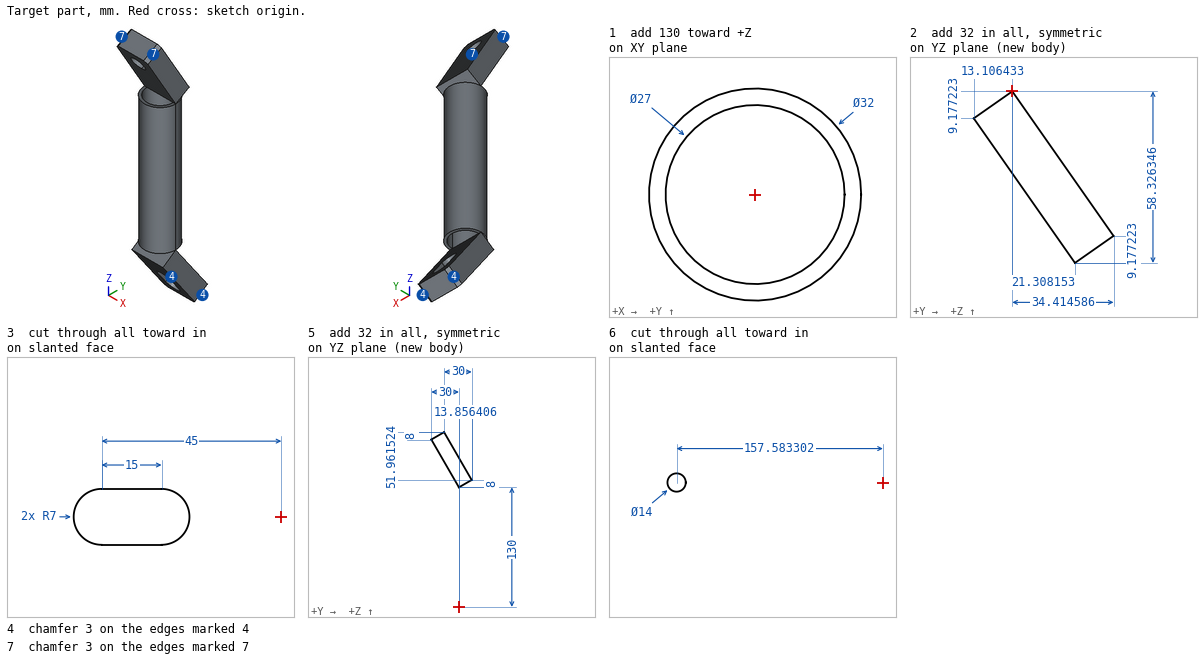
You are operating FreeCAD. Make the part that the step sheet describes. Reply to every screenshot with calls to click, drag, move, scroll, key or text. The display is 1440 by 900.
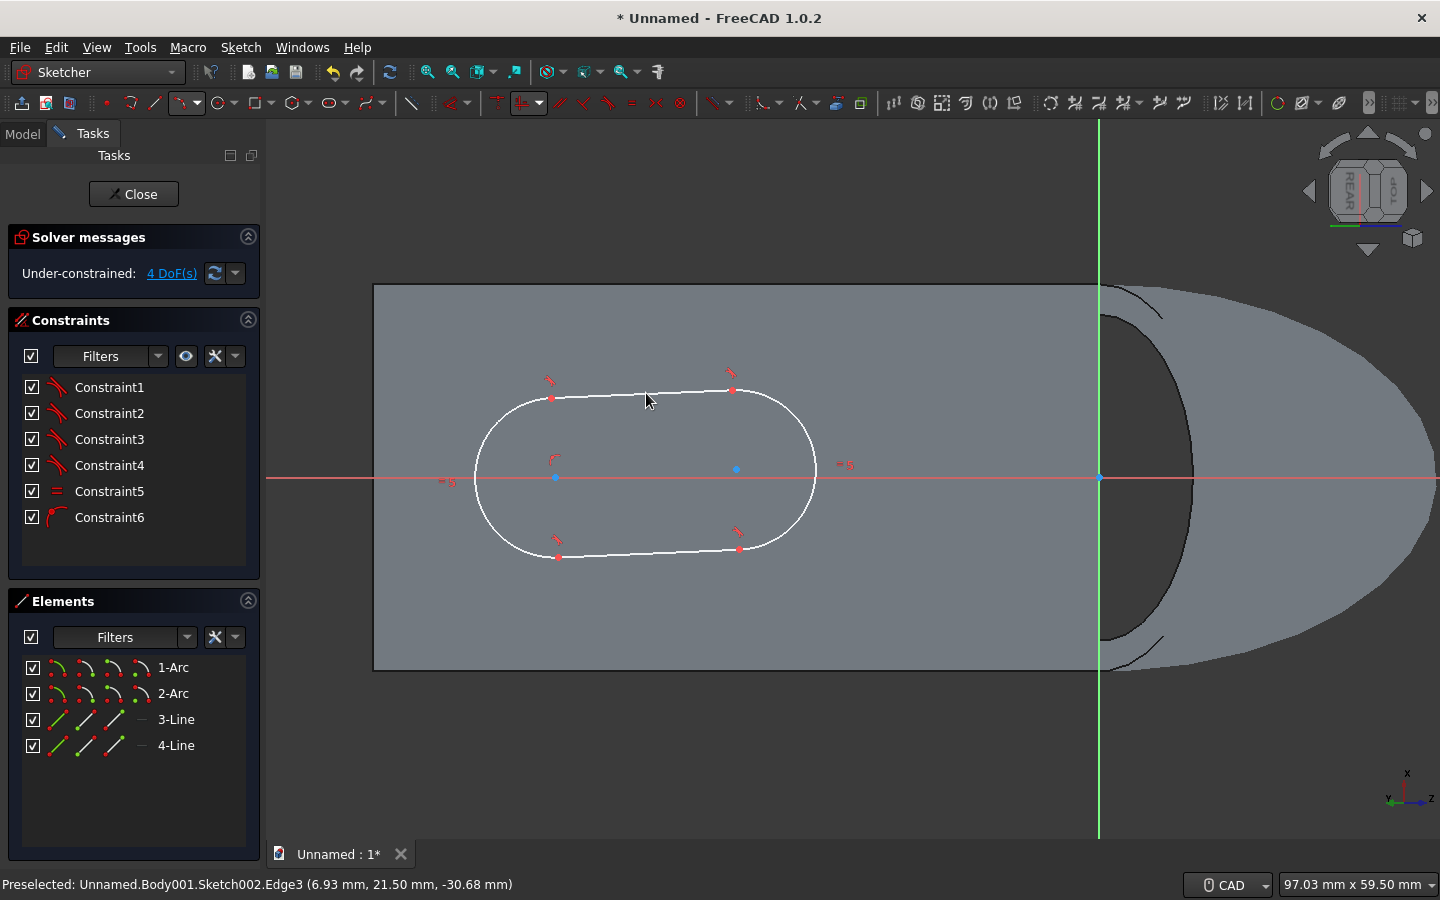
click(606, 396)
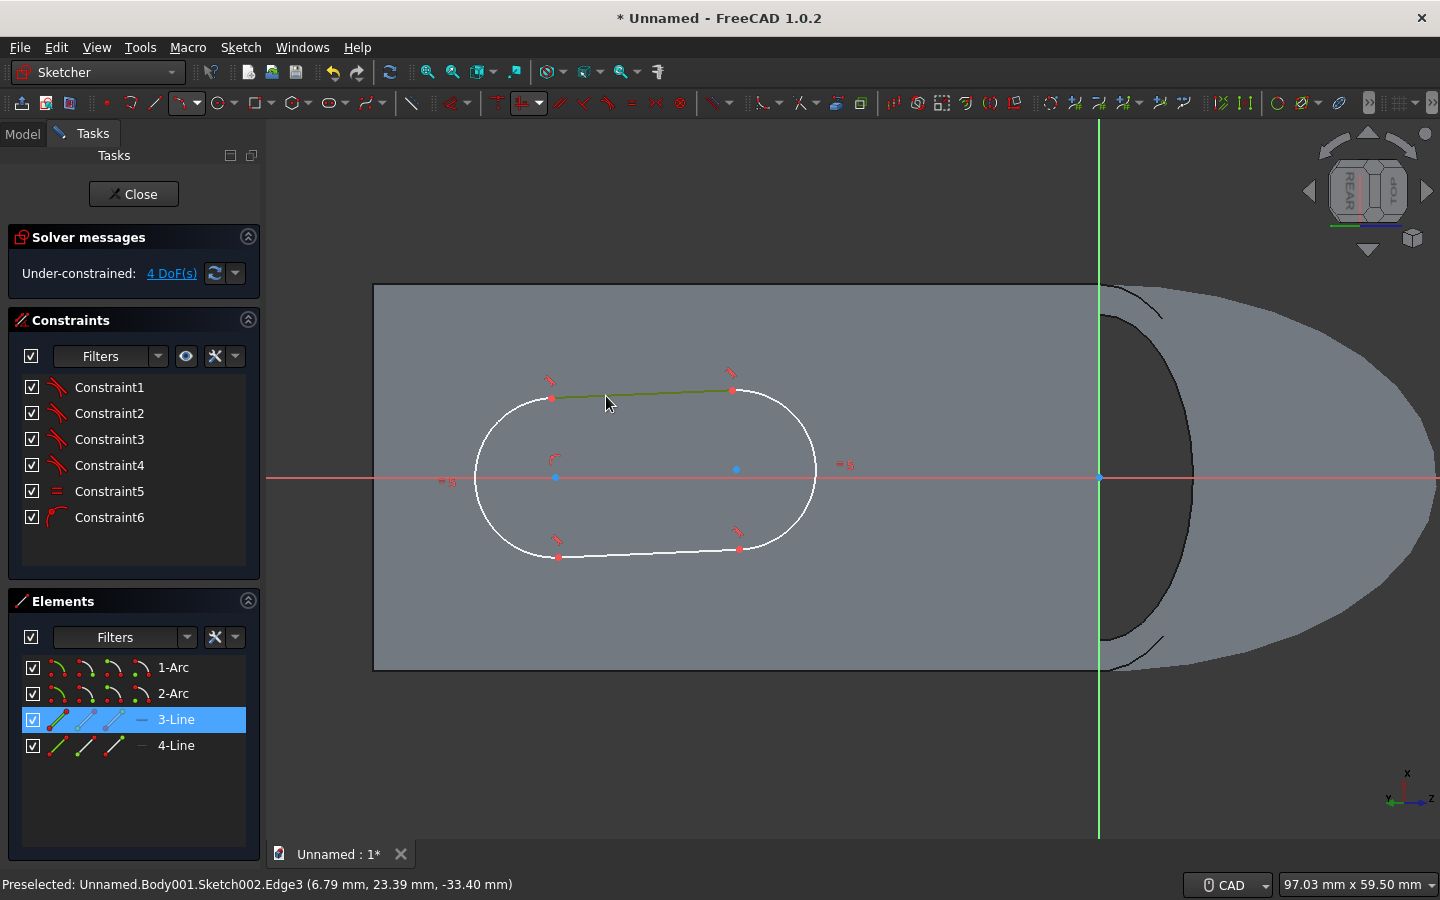
key(h)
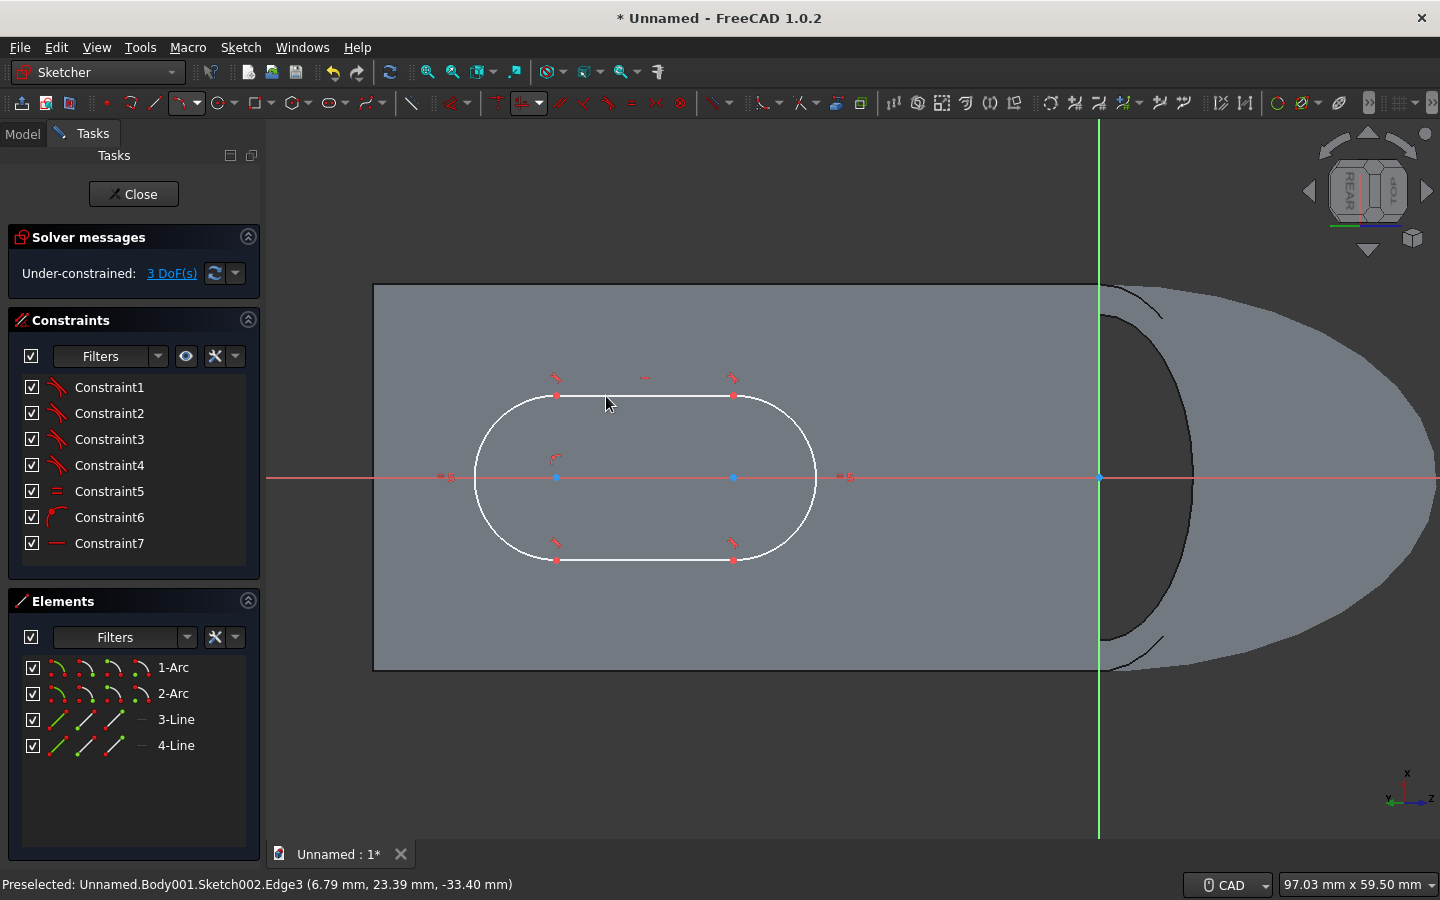
click(450, 104)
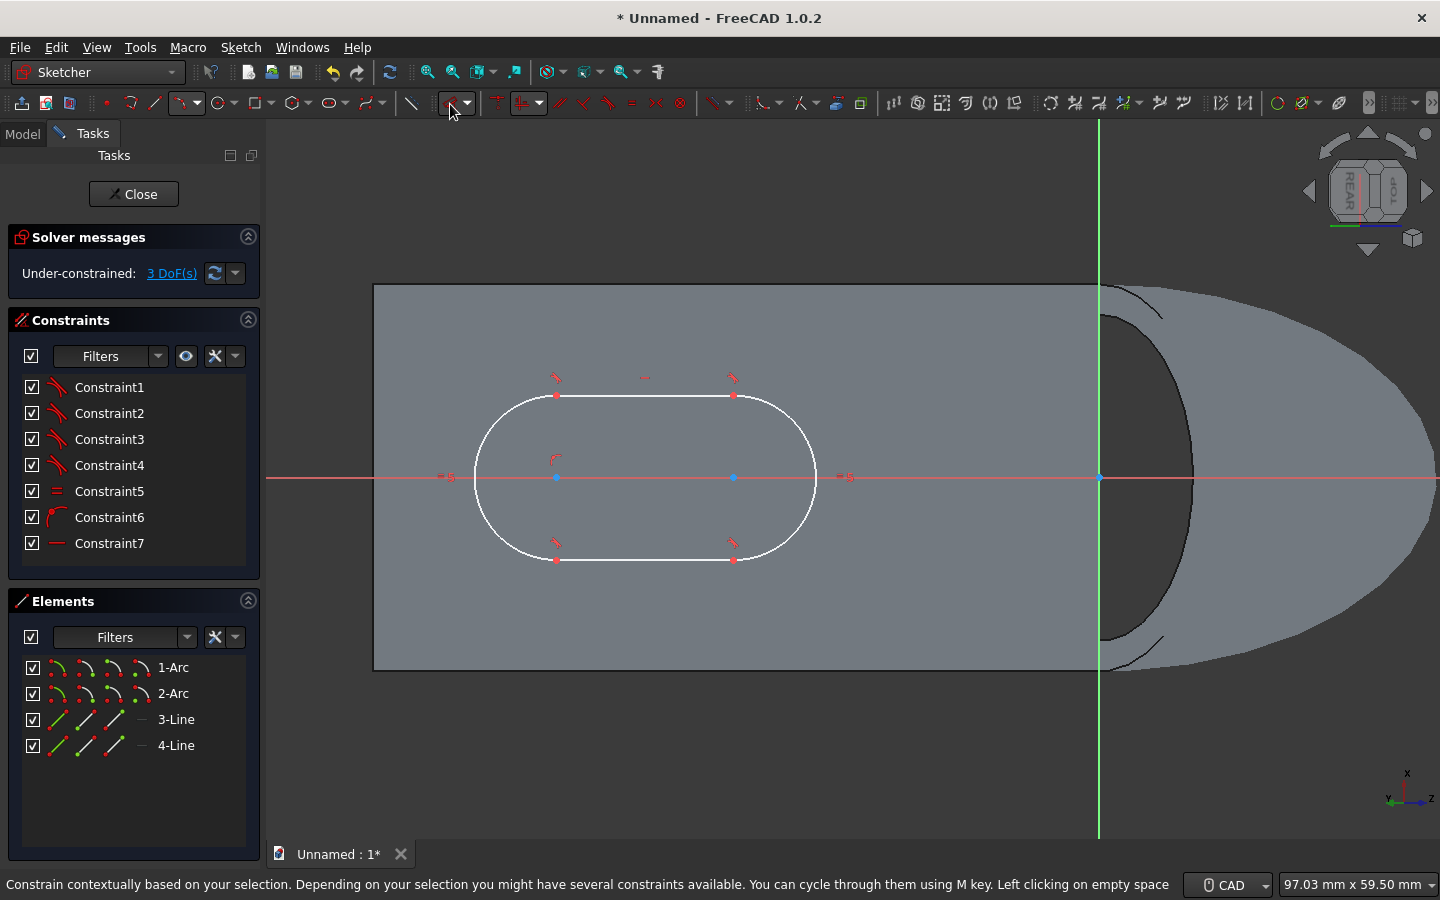
click(490, 430)
click(464, 411)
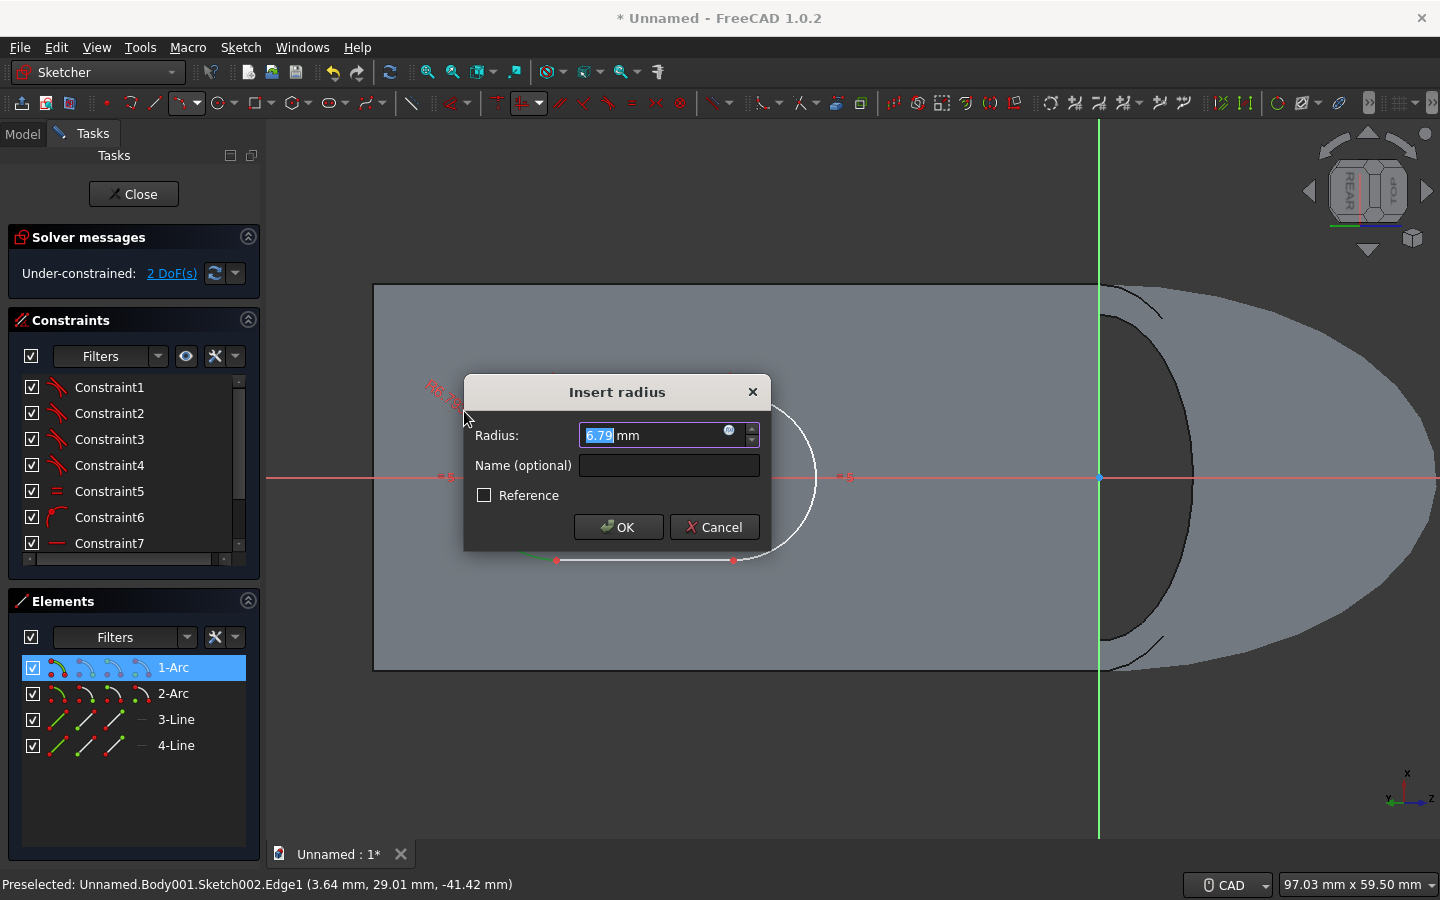
text(7)
key(Return)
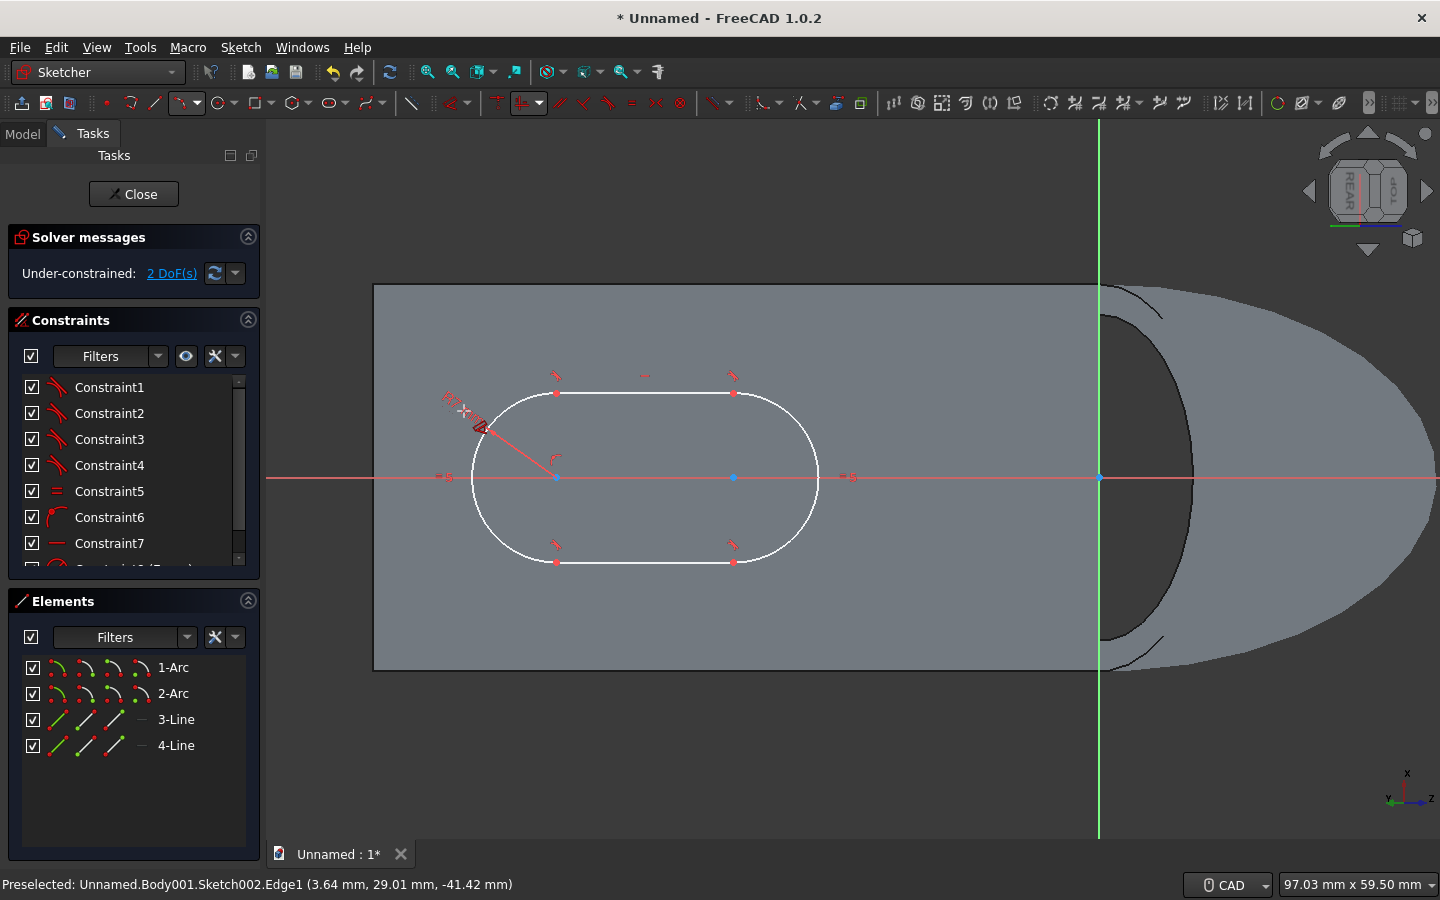
click(610, 393)
click(645, 359)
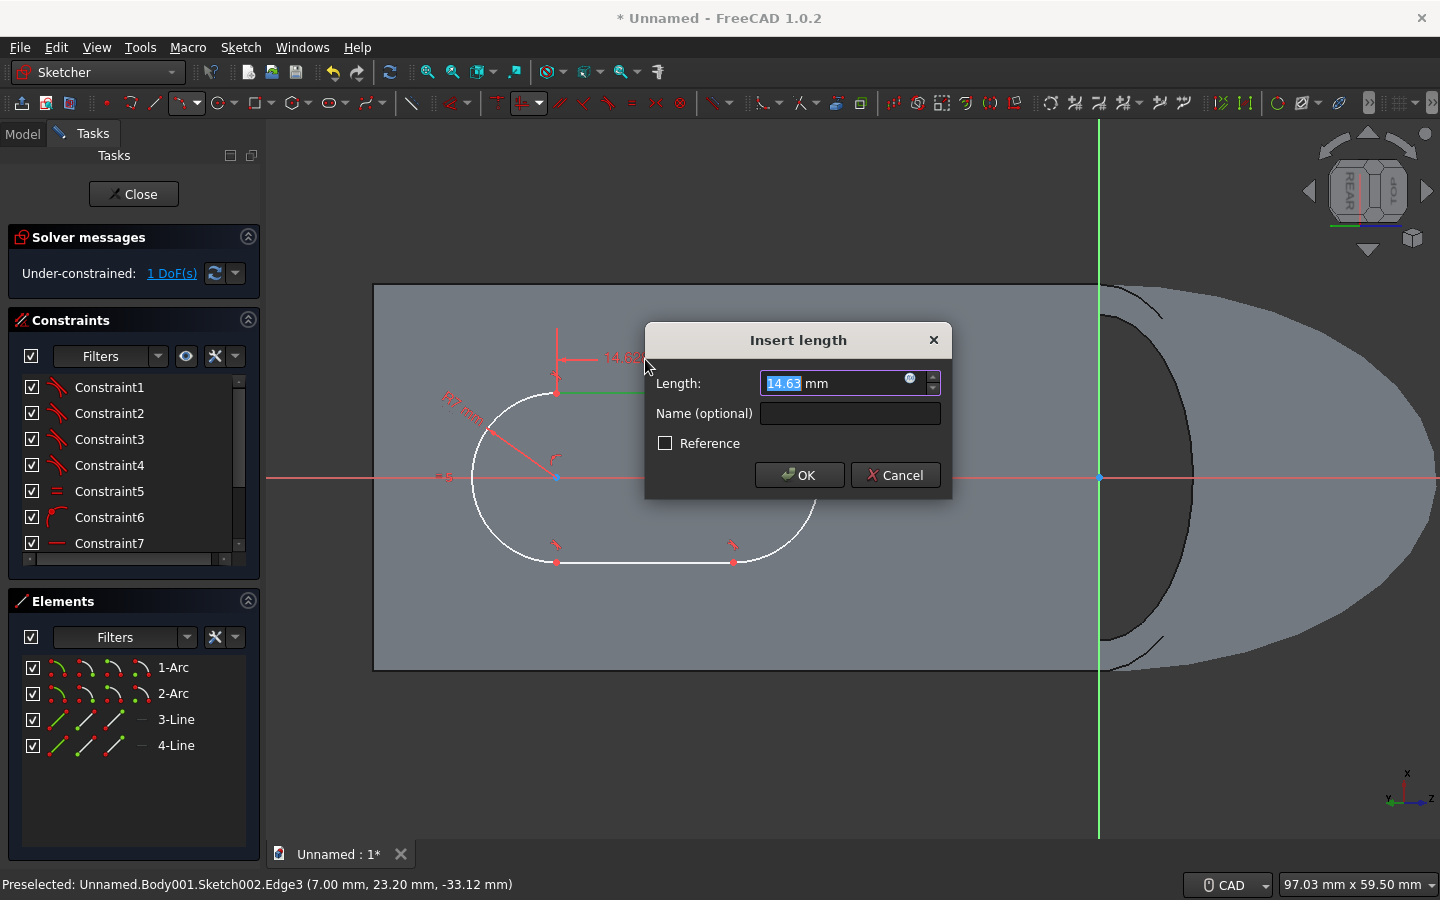
text(15)
key(Return)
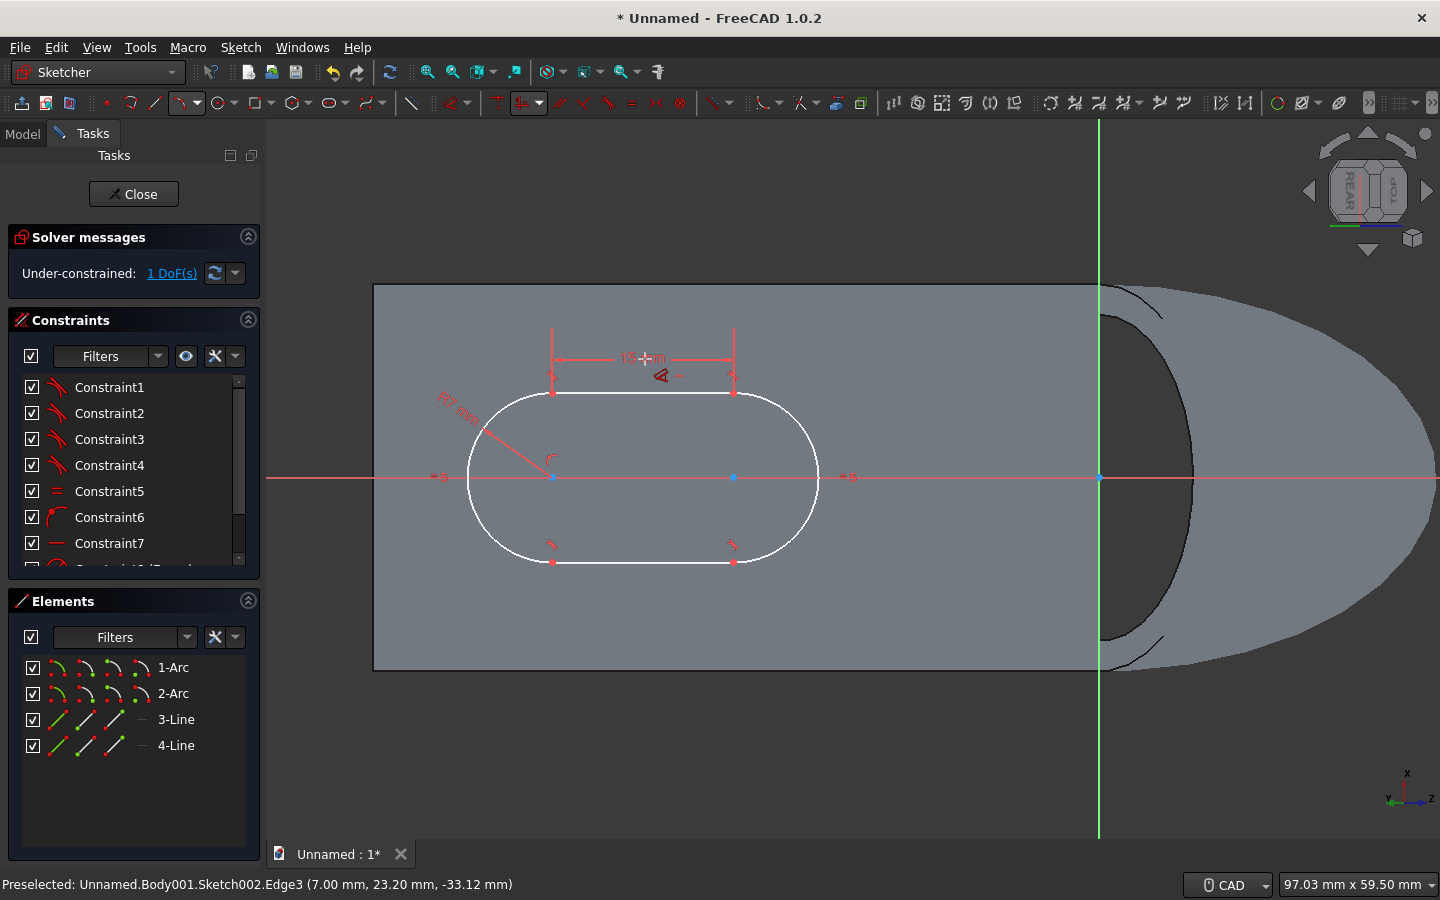
click(552, 393)
click(826, 359)